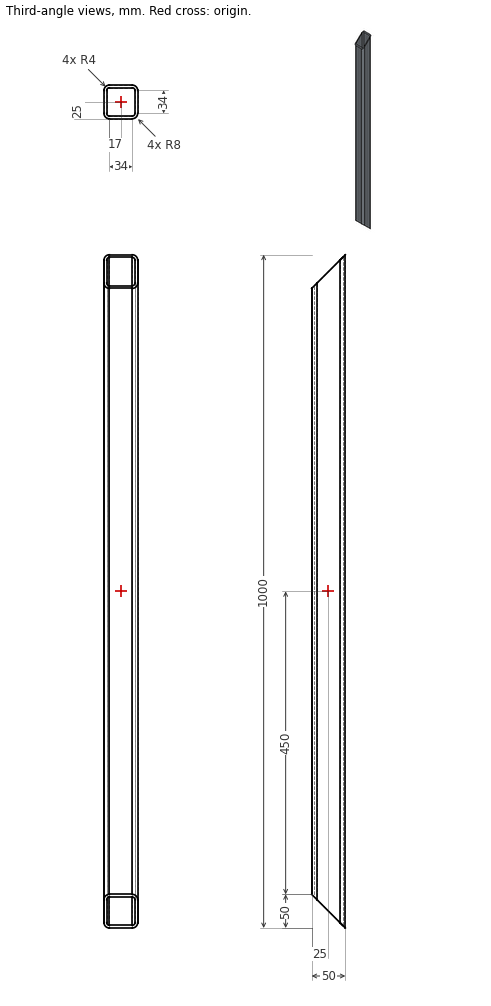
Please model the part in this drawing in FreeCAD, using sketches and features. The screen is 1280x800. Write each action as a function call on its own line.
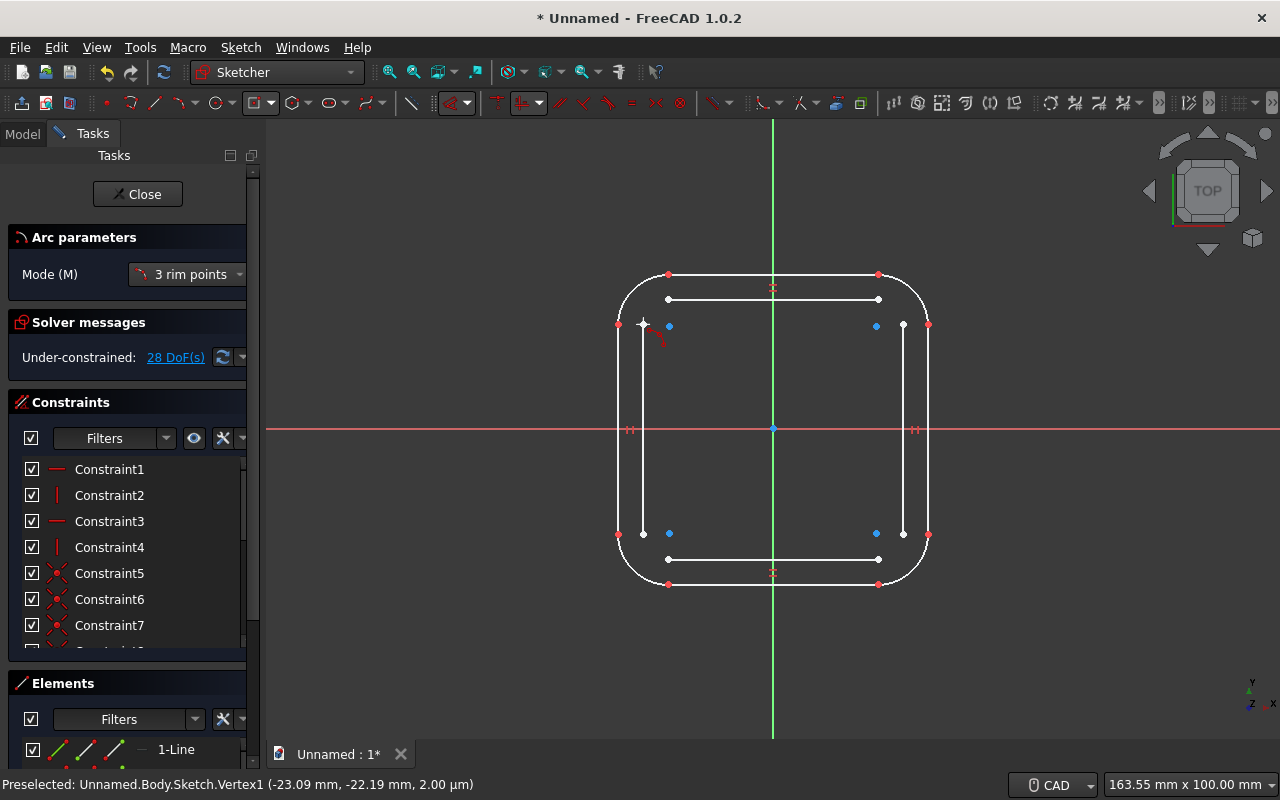
click(878, 300)
click(903, 325)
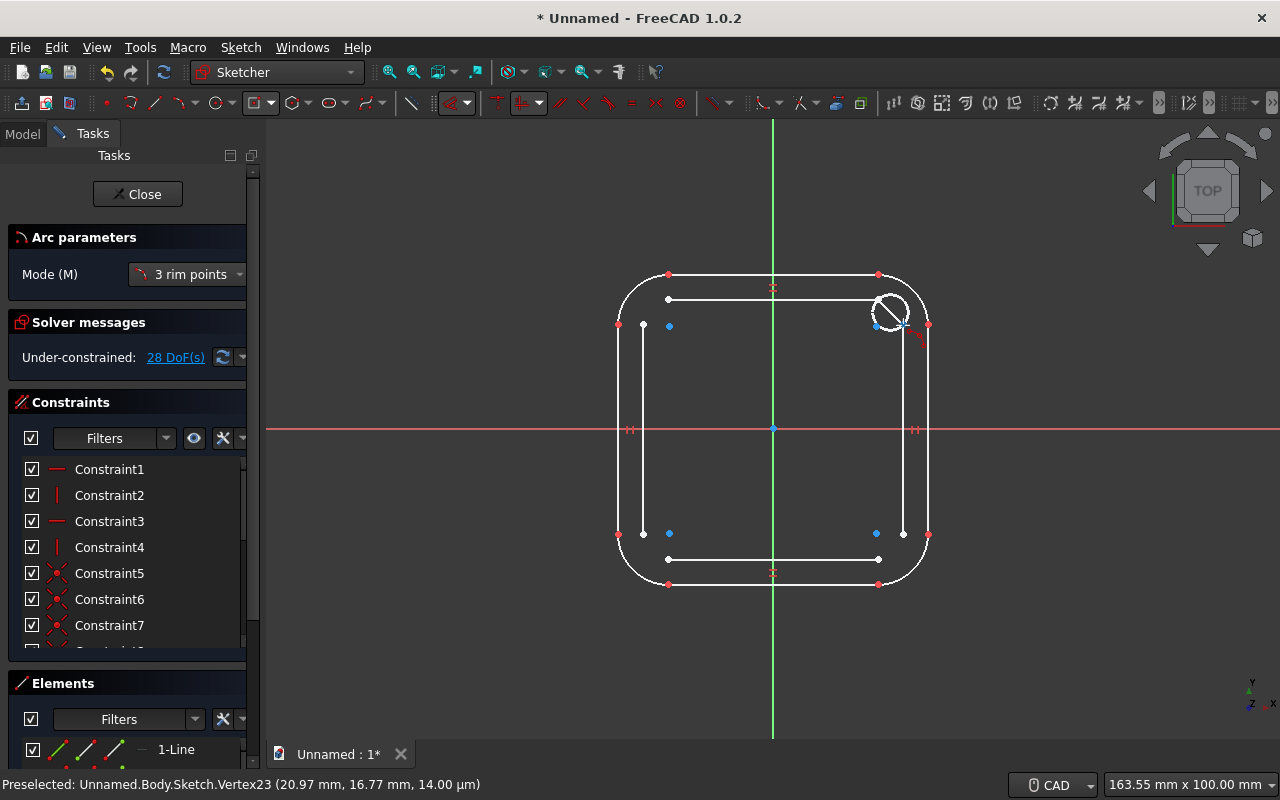
scroll(896, 306, up, 4)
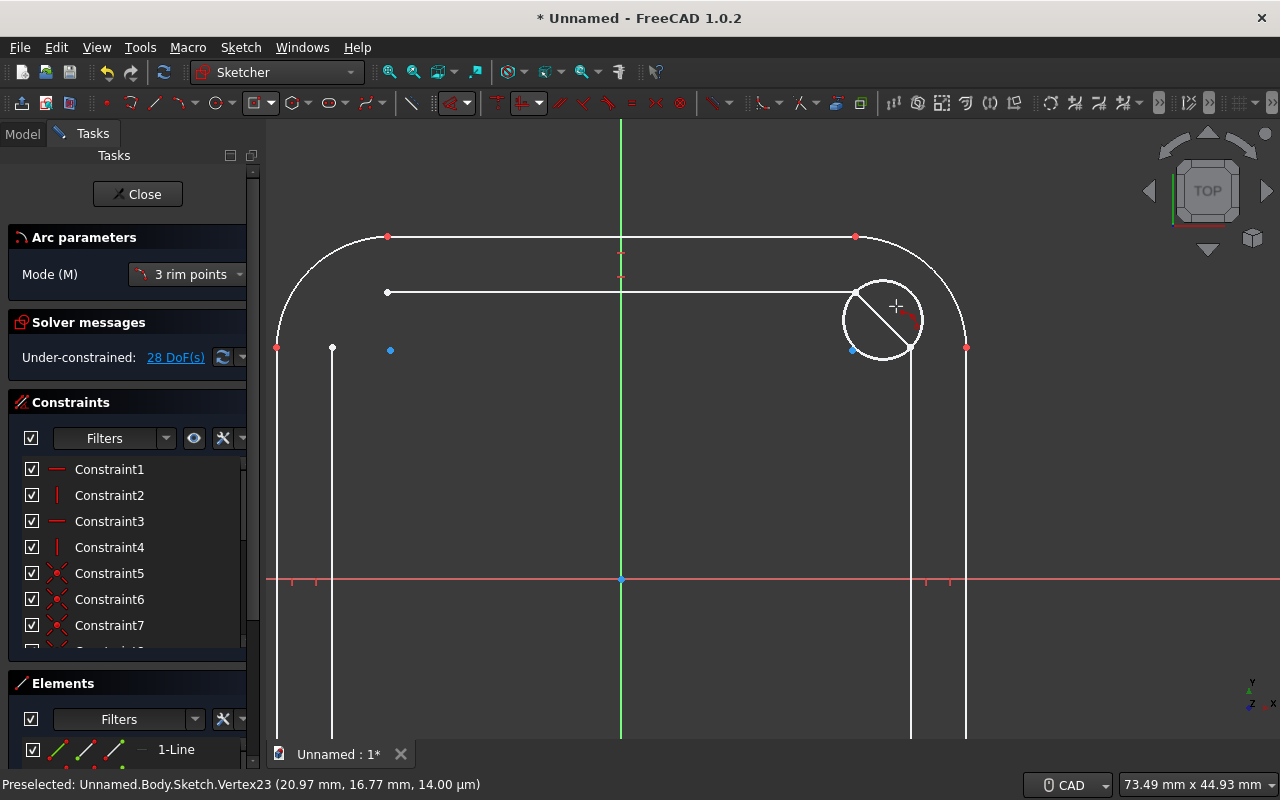
click(895, 306)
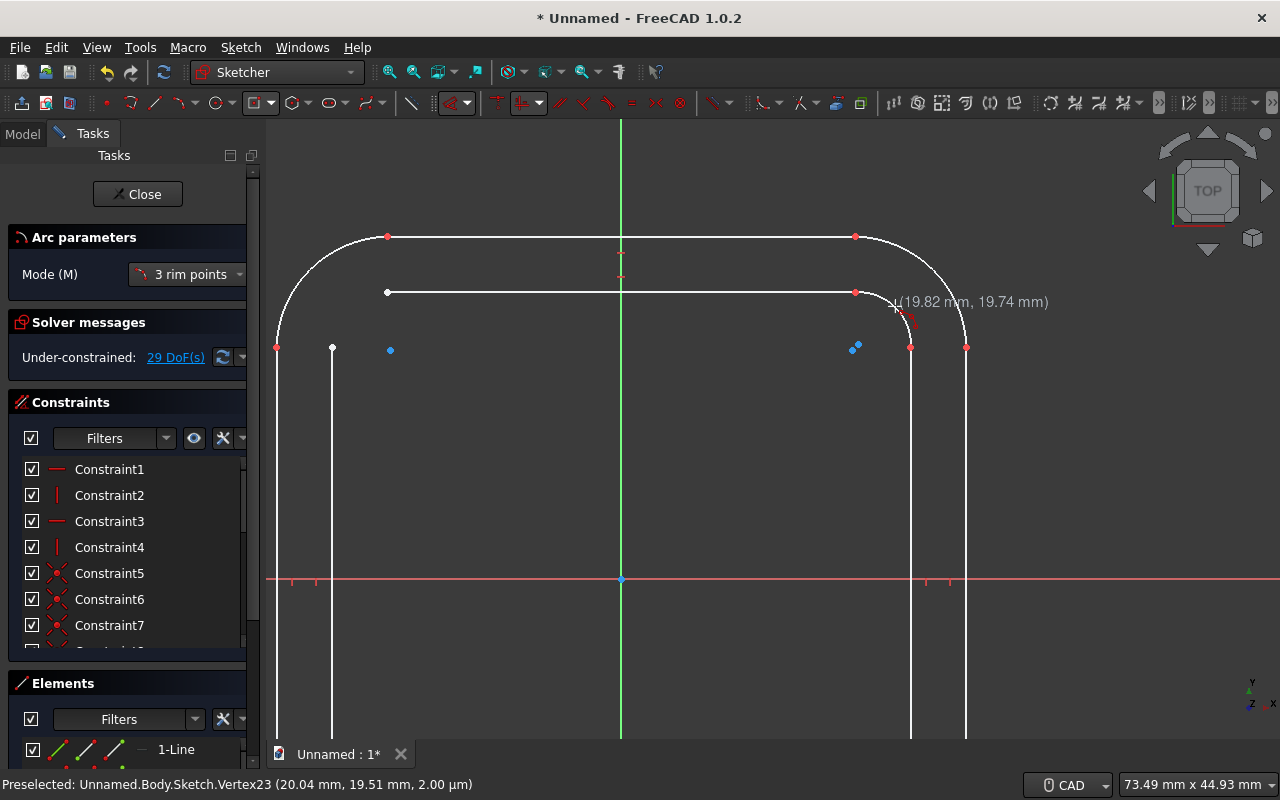
scroll(805, 246, down, 3)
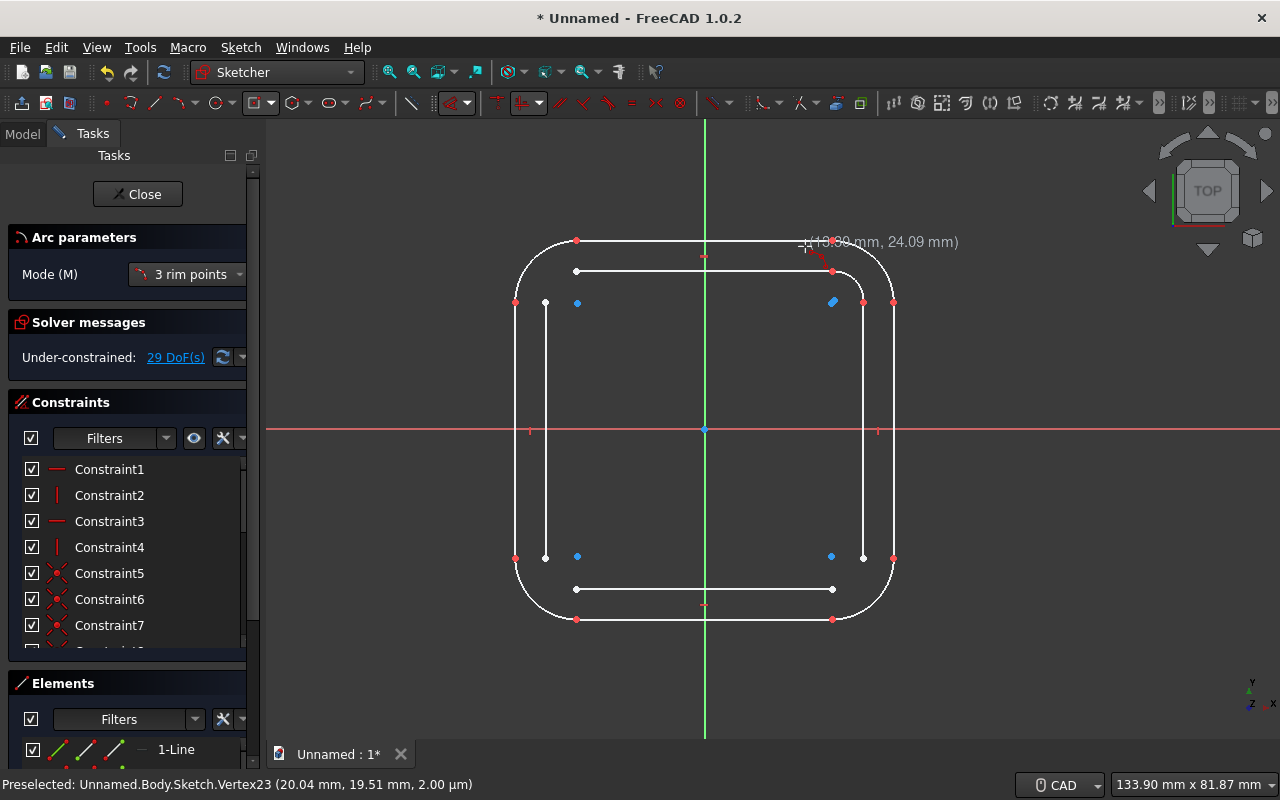
click(863, 559)
click(833, 589)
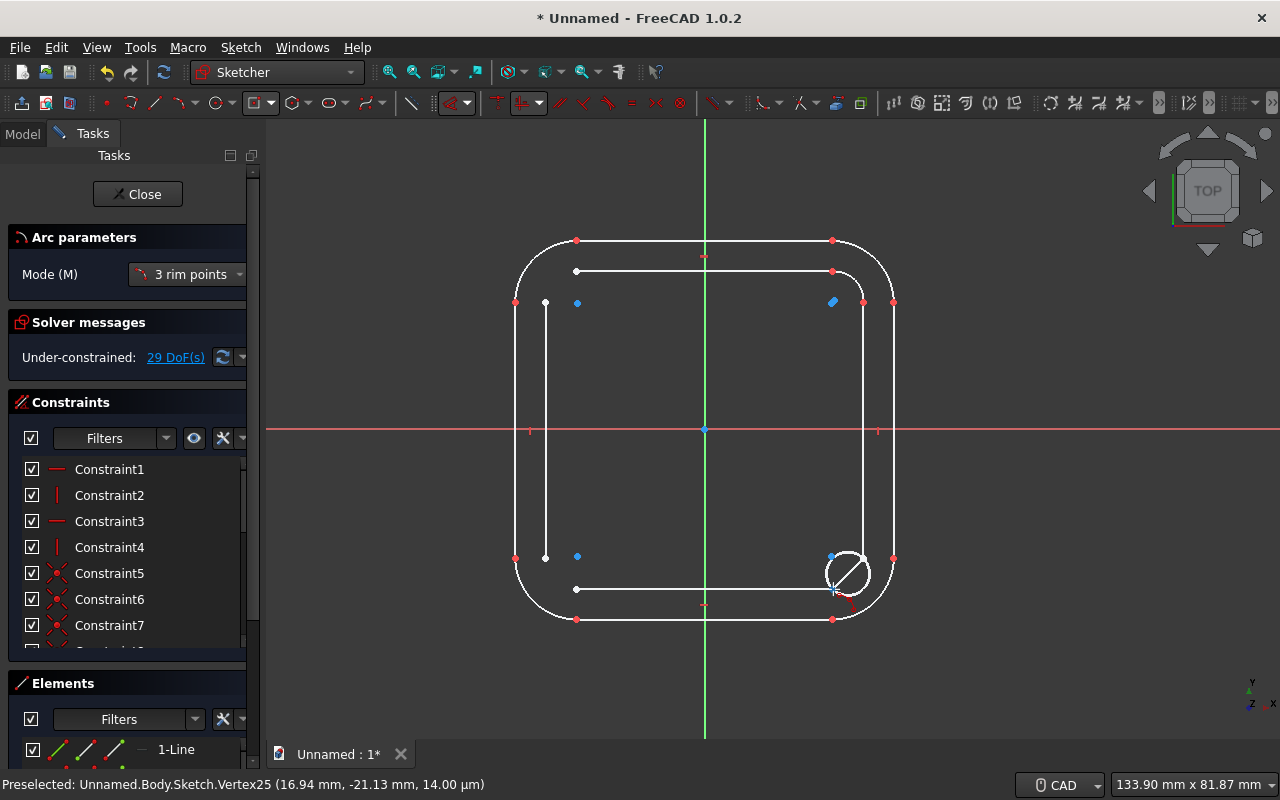
scroll(855, 579, up, 3)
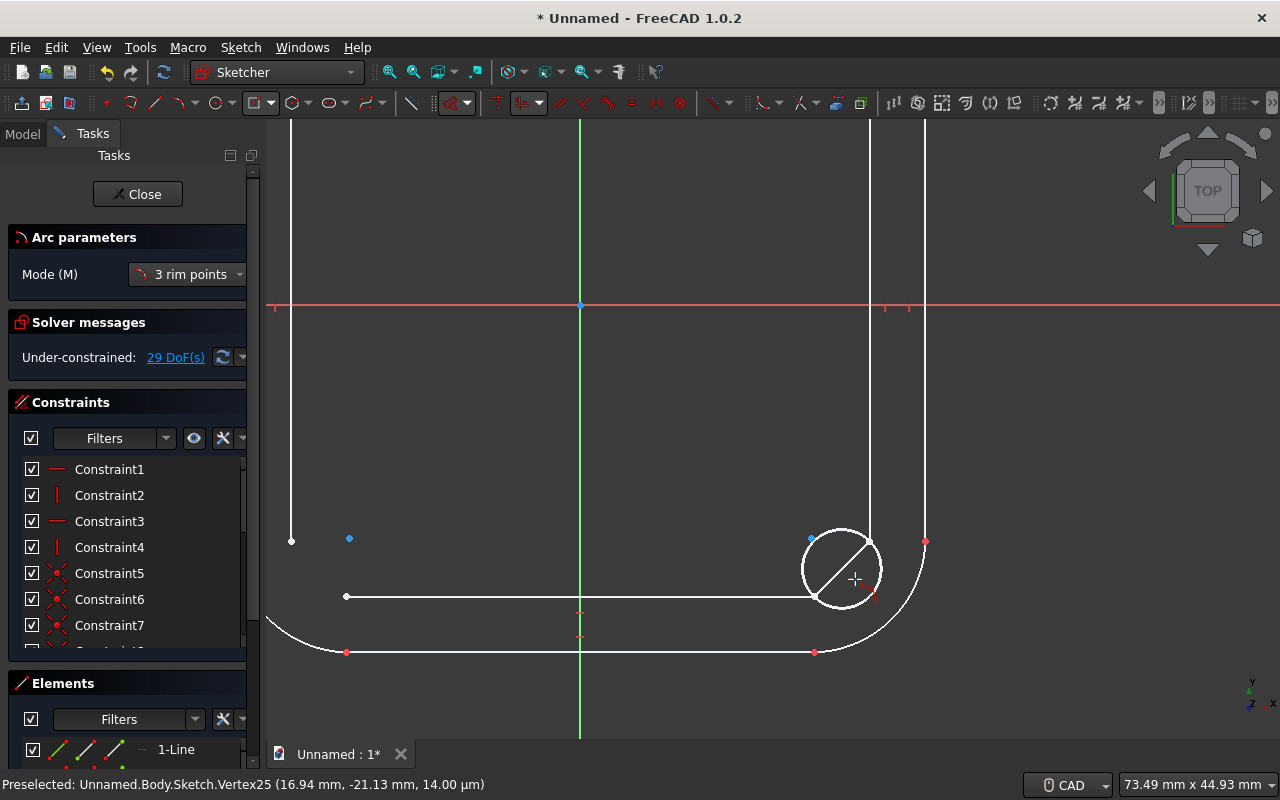
click(854, 579)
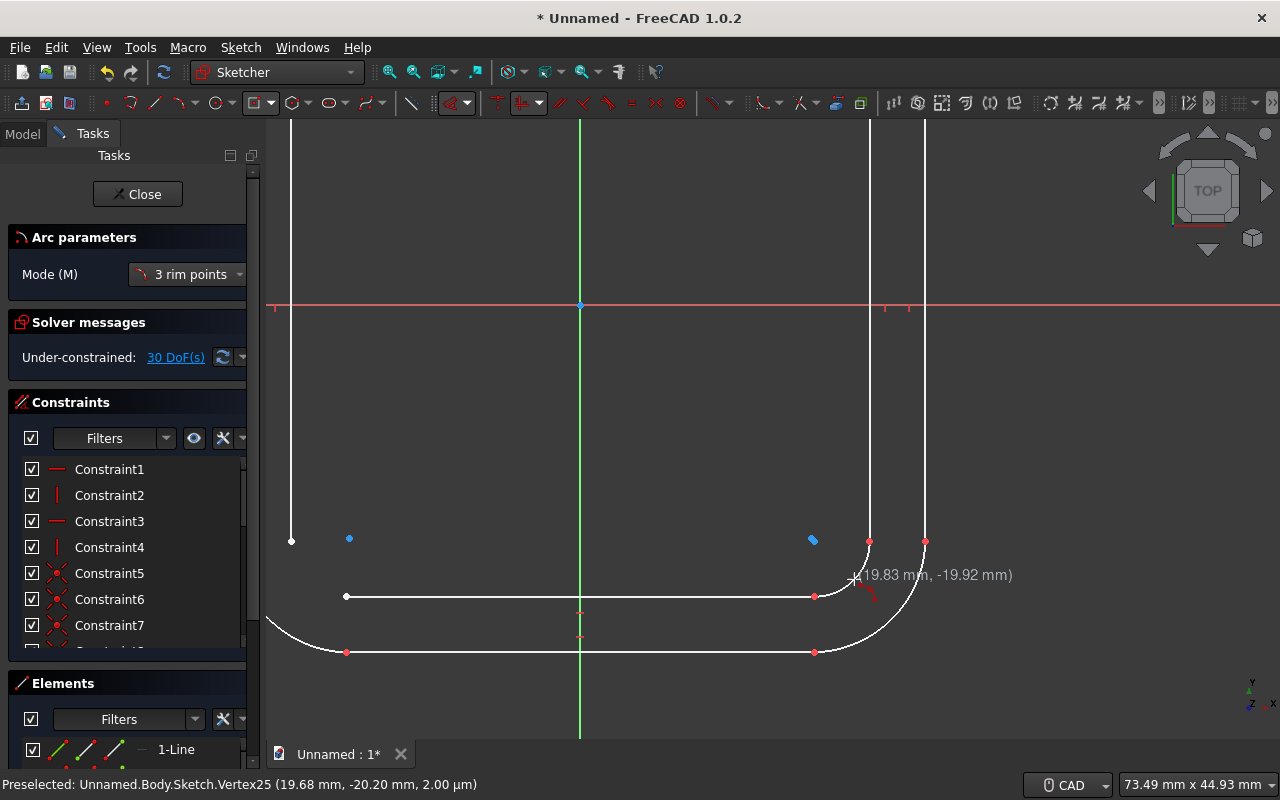
click(347, 597)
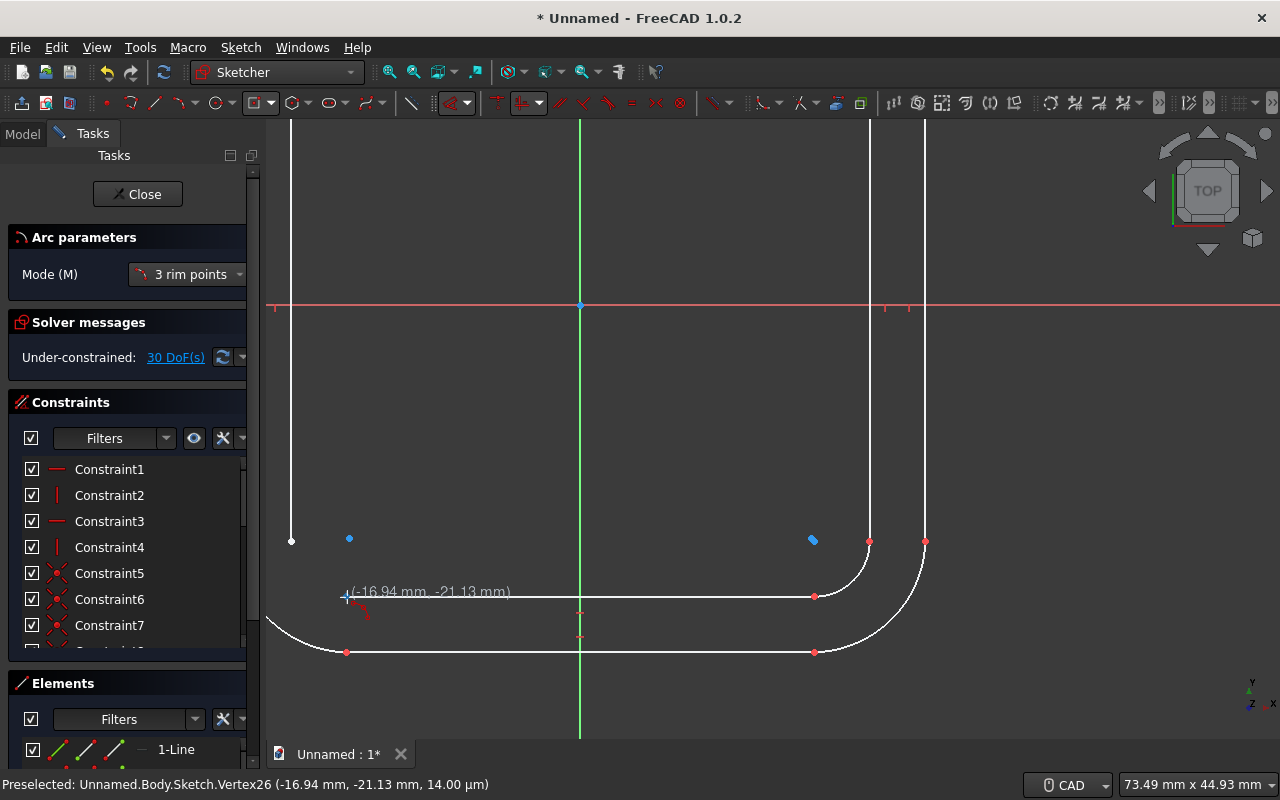
scroll(856, 580, down, 3)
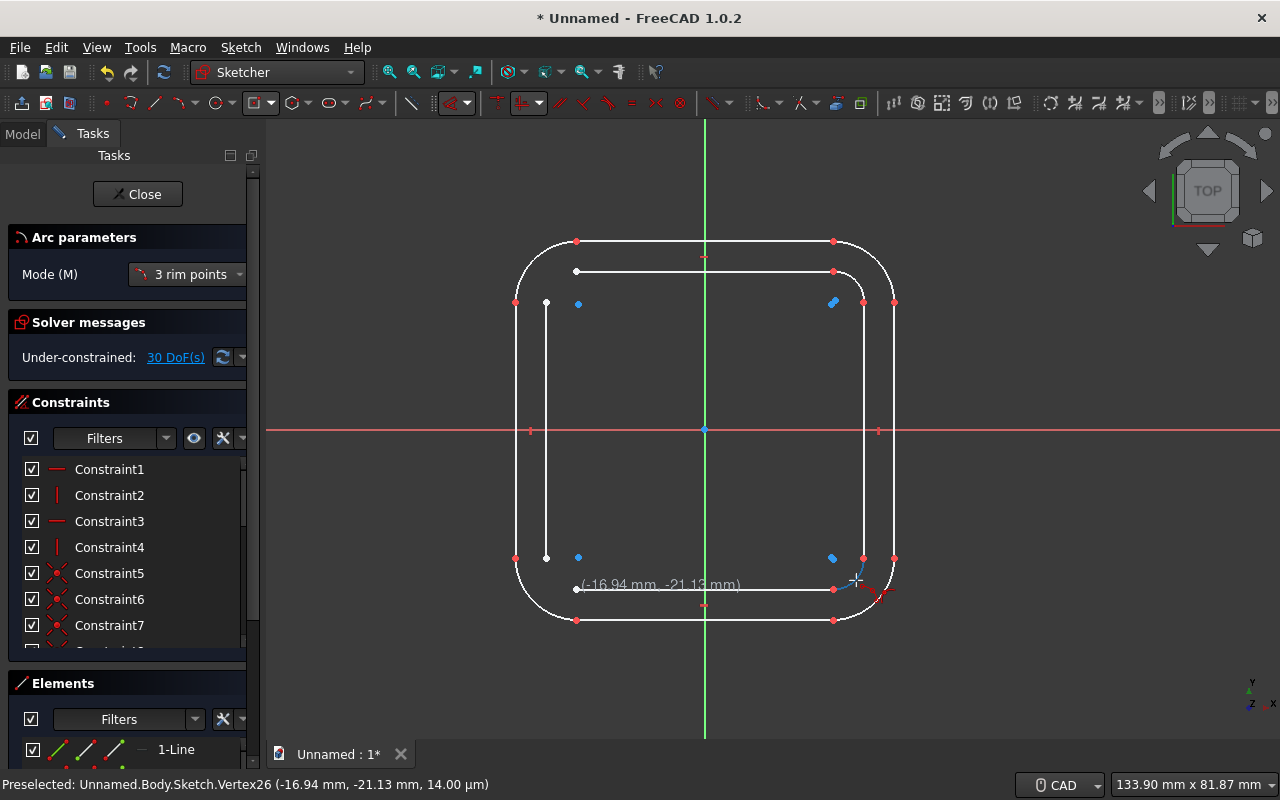
click(546, 559)